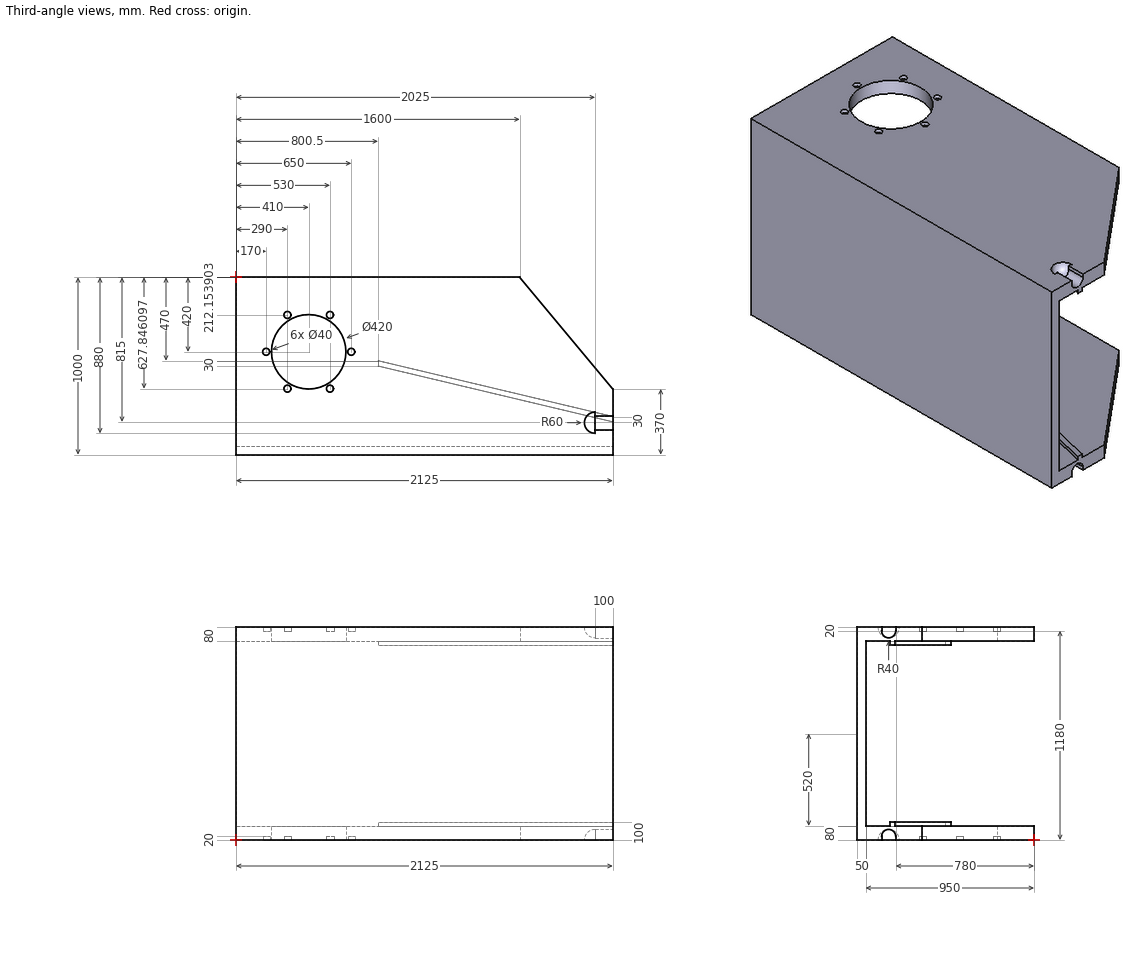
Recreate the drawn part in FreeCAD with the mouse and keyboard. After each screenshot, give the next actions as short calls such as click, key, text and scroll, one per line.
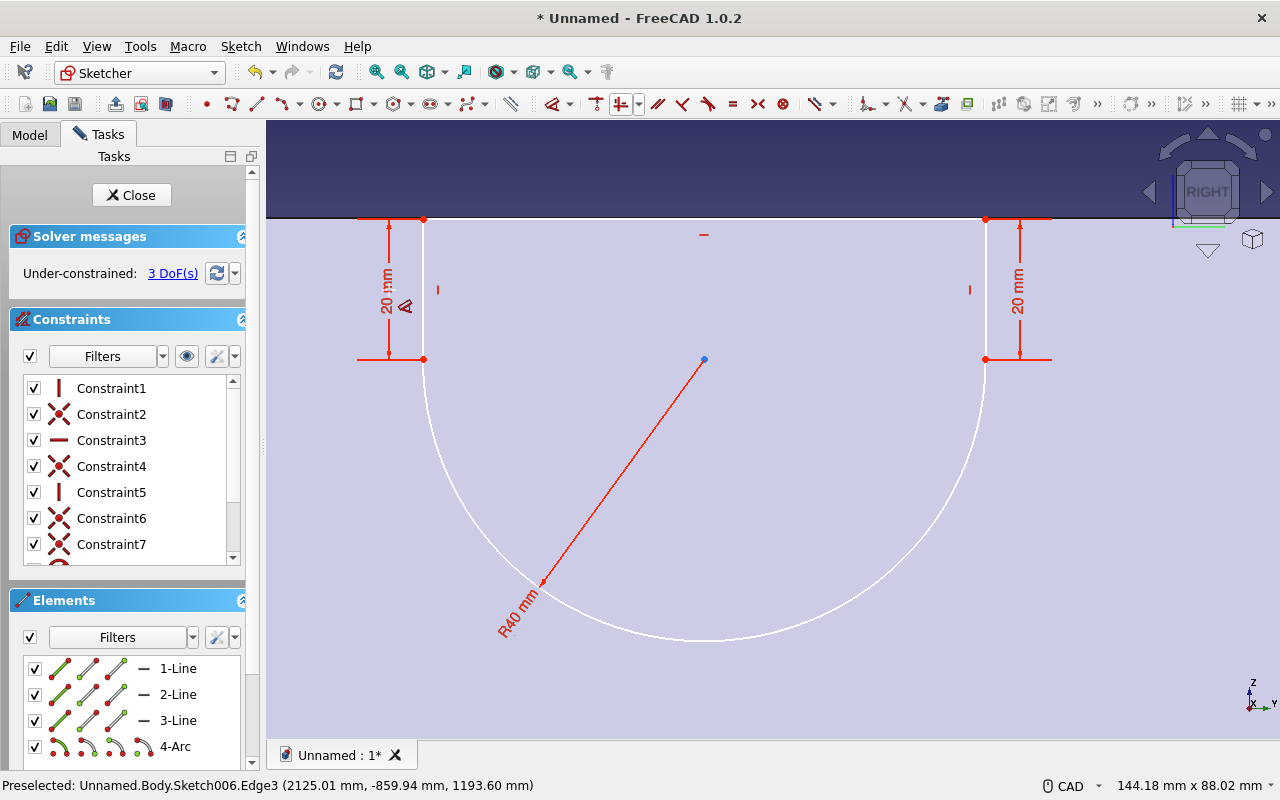
click(986, 360)
click(1050, 326)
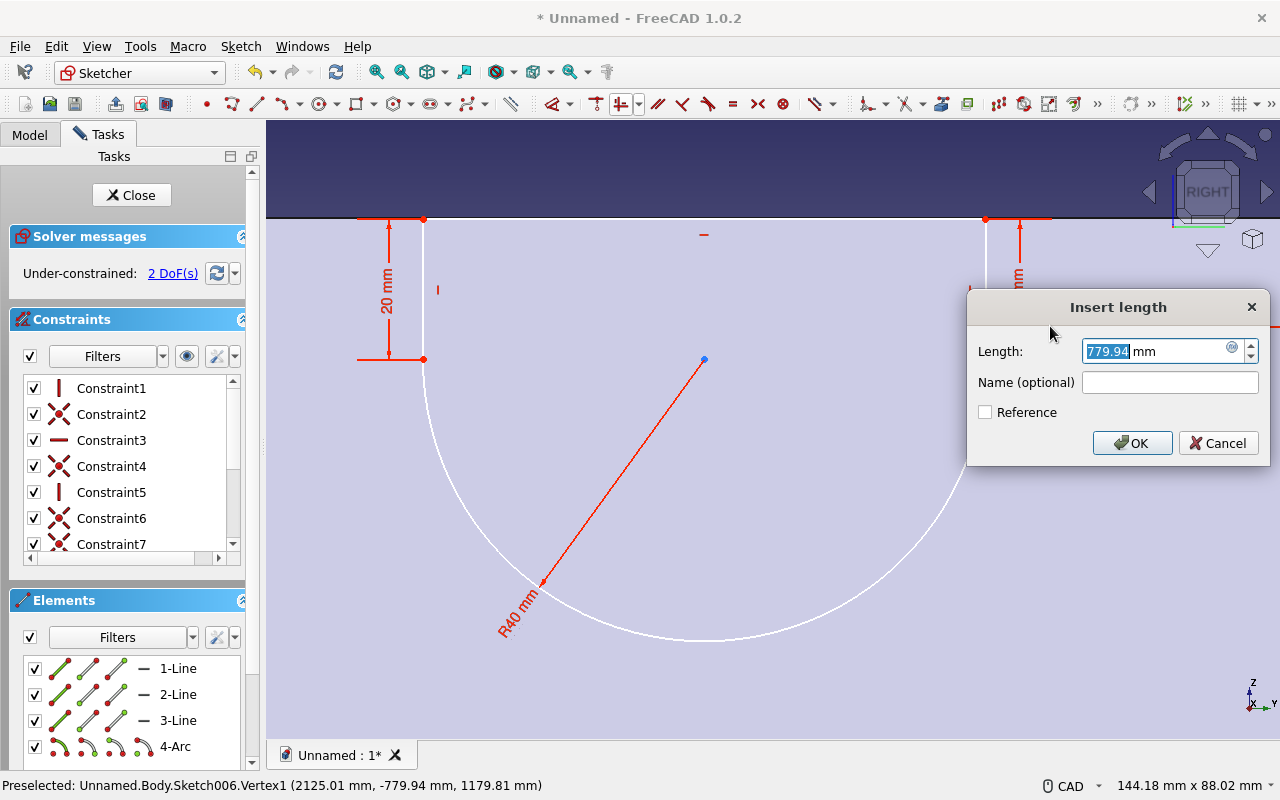
text(780)
key(Return)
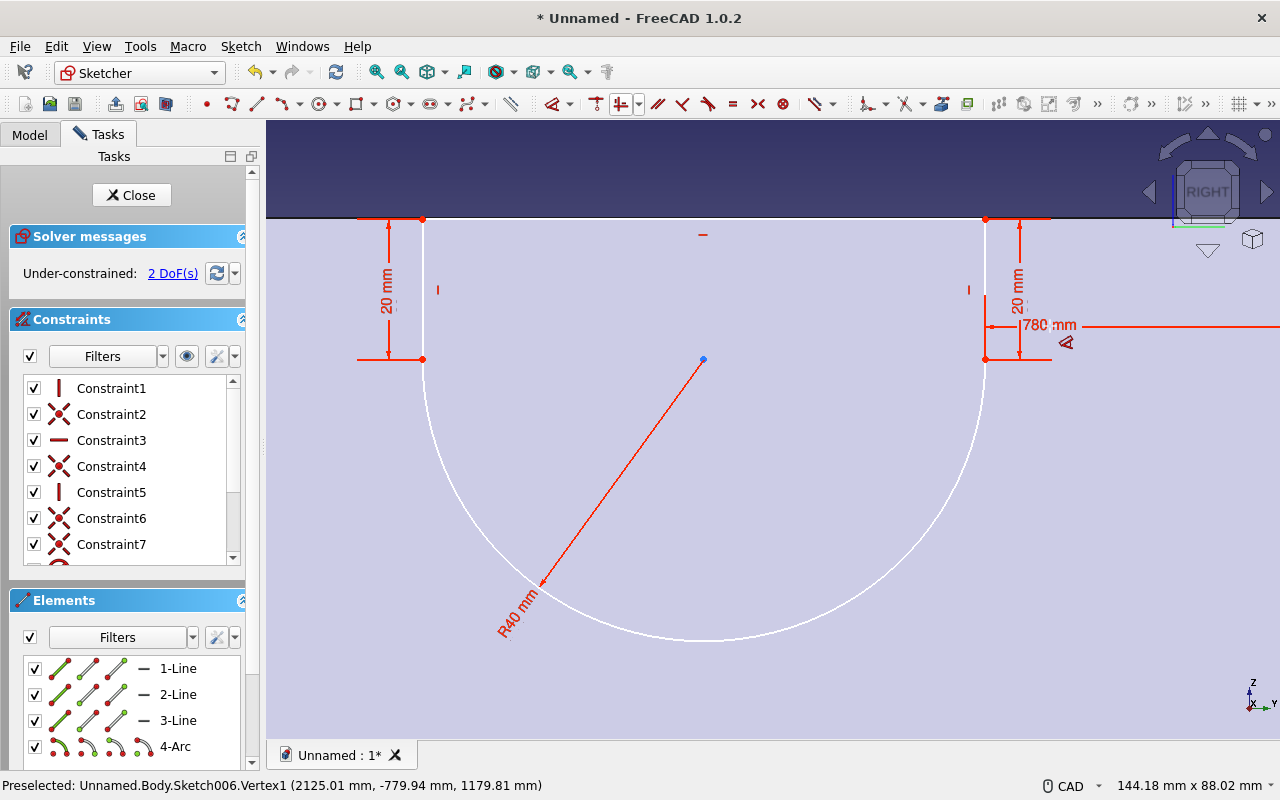
click(985, 360)
click(951, 536)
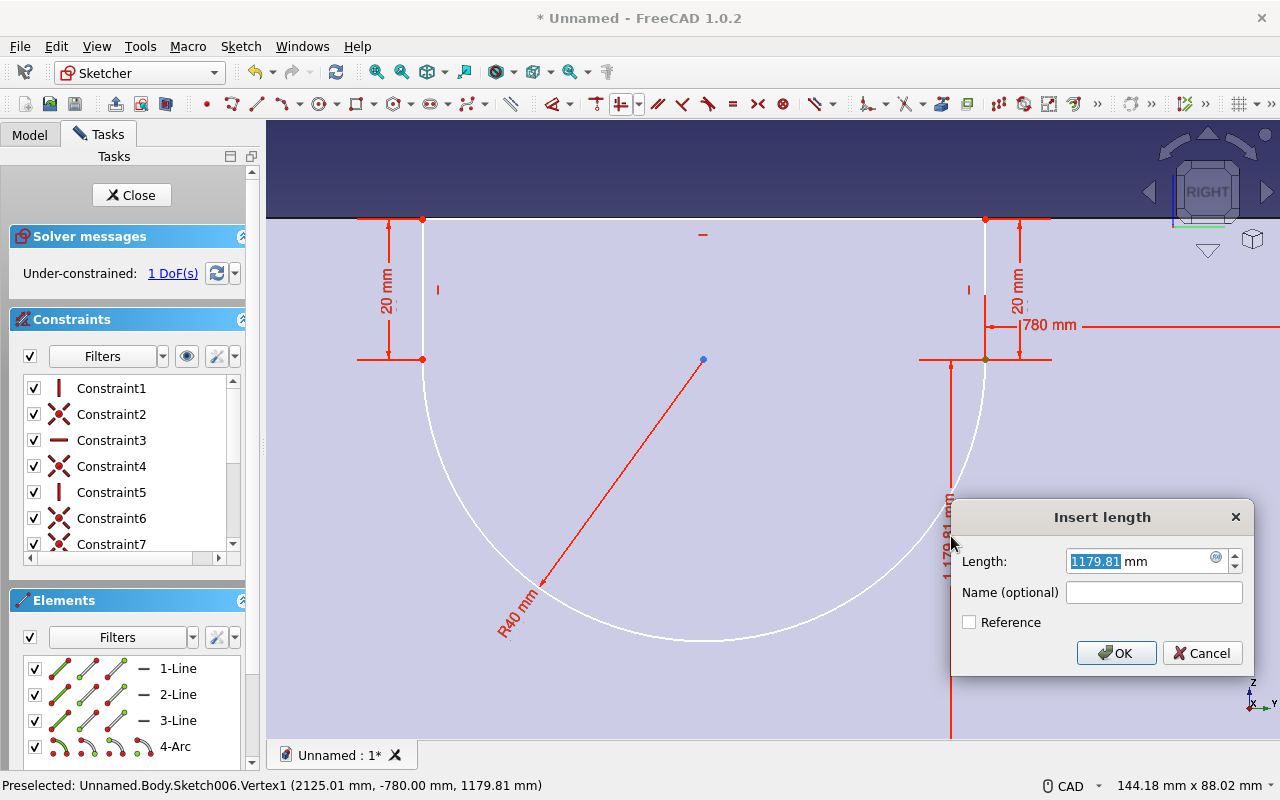
text(1180)
key(Return)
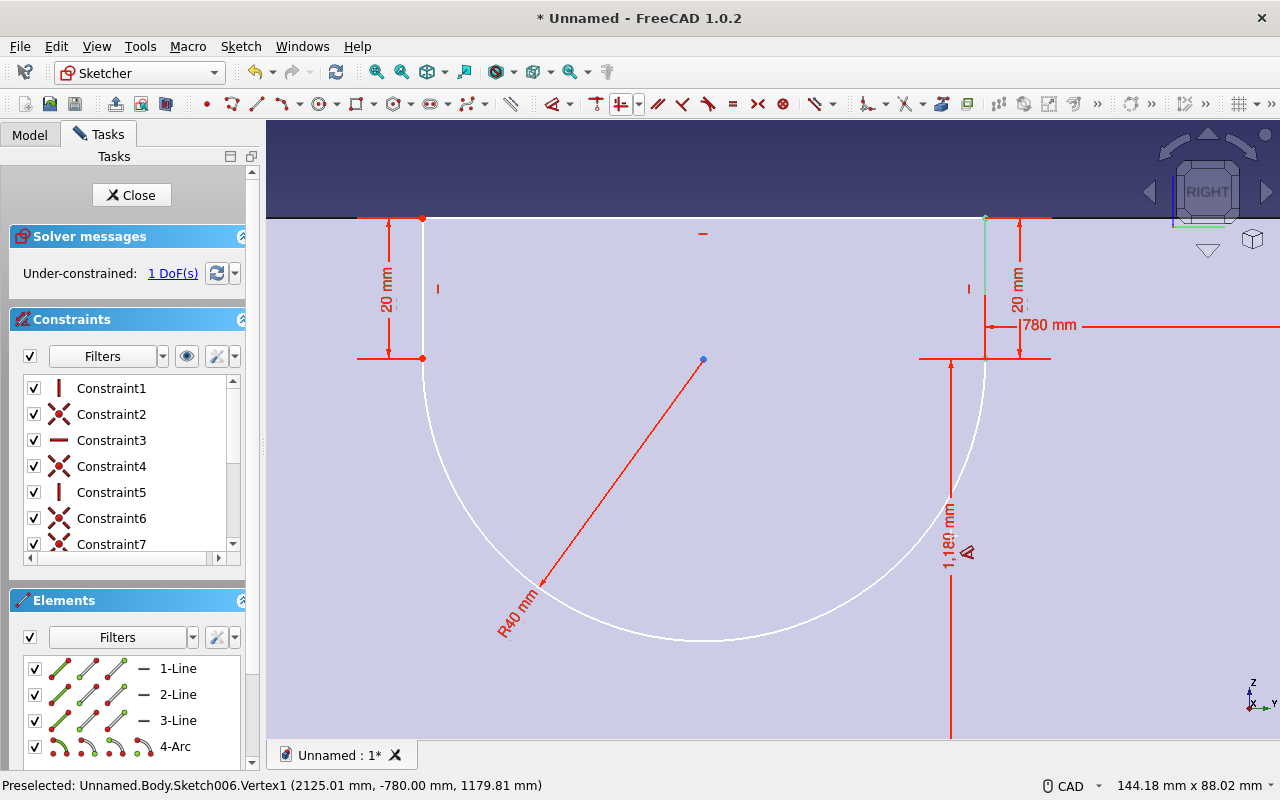
click(704, 360)
click(670, 536)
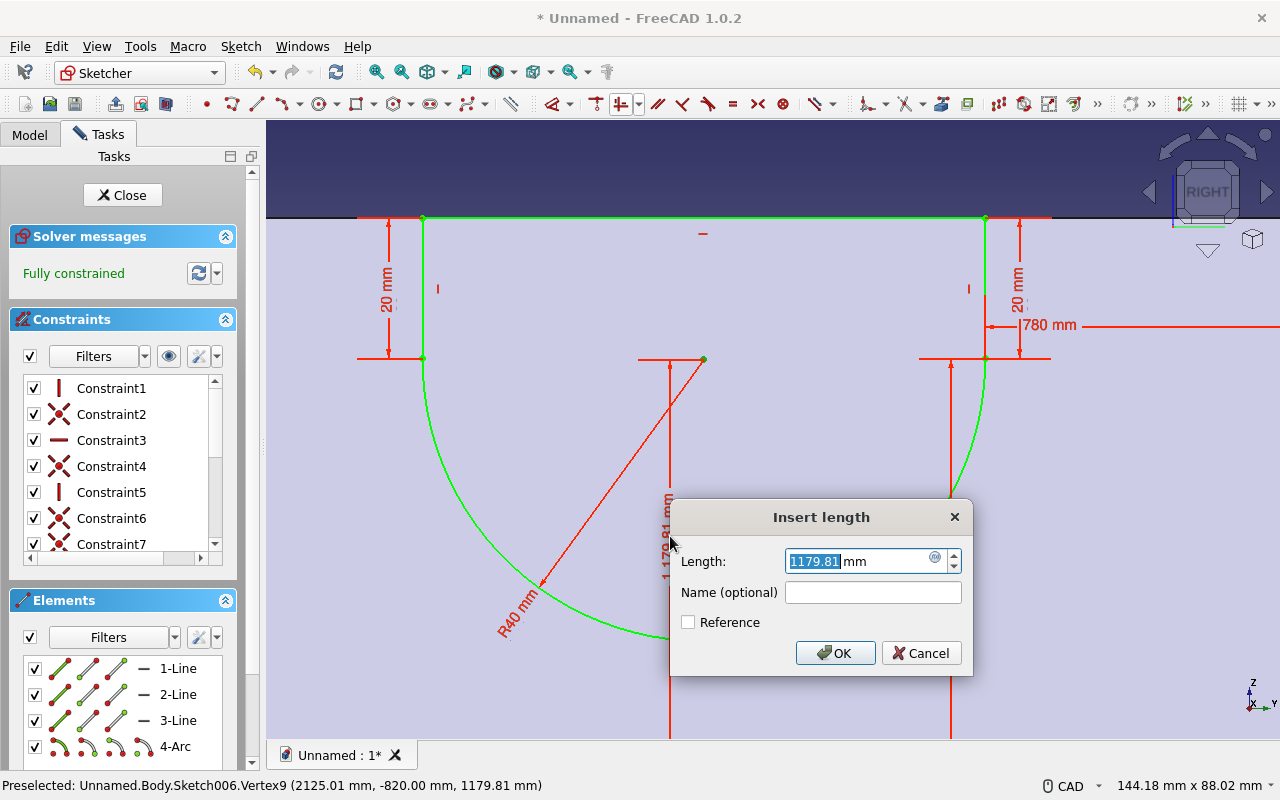
text(1180)
key(Return)
key(Escape)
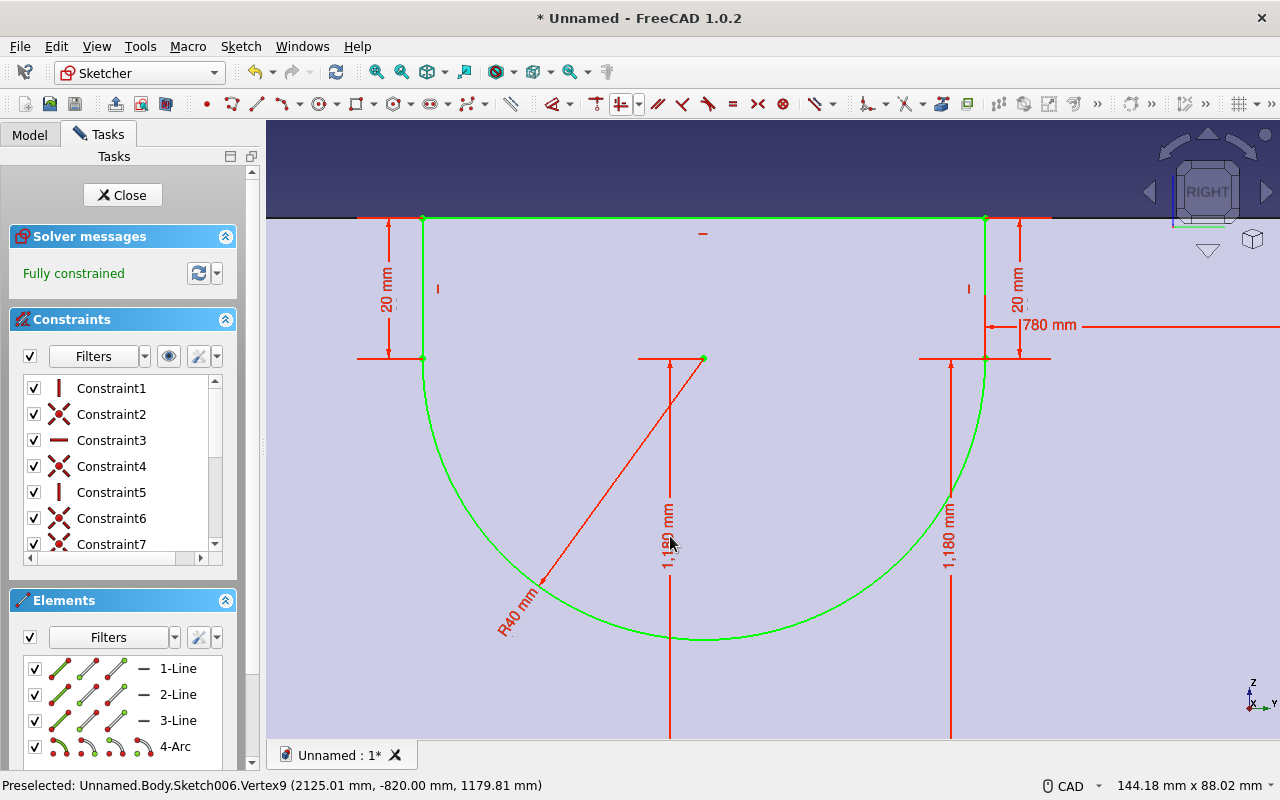
click(123, 195)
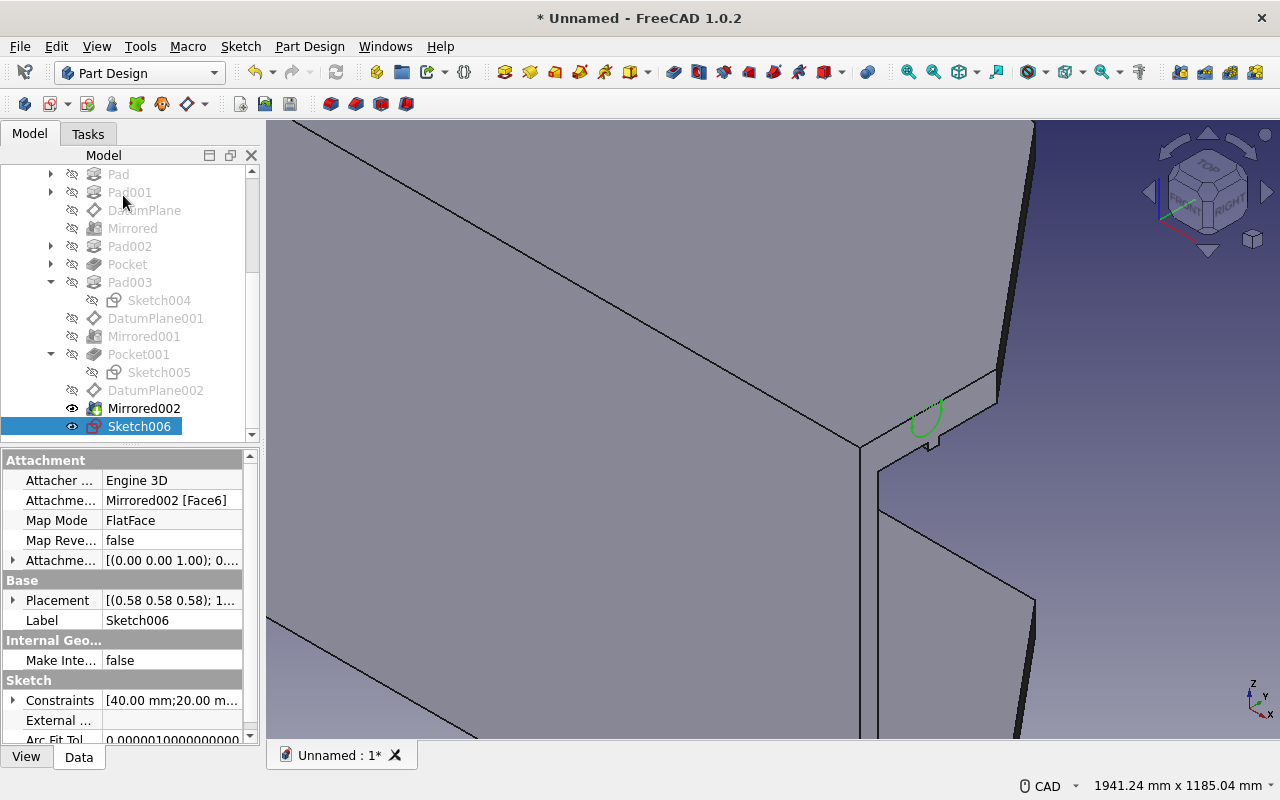
click(674, 72)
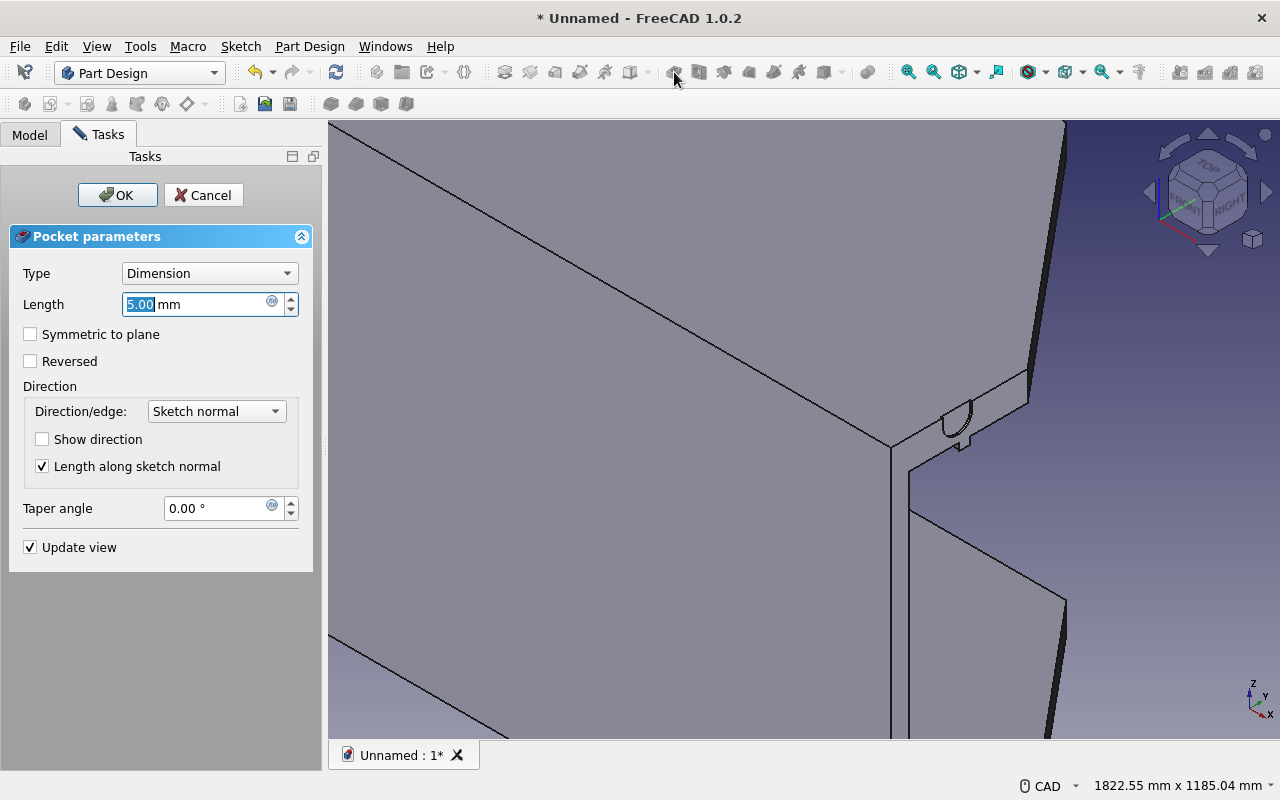
text(100)
key(Tab)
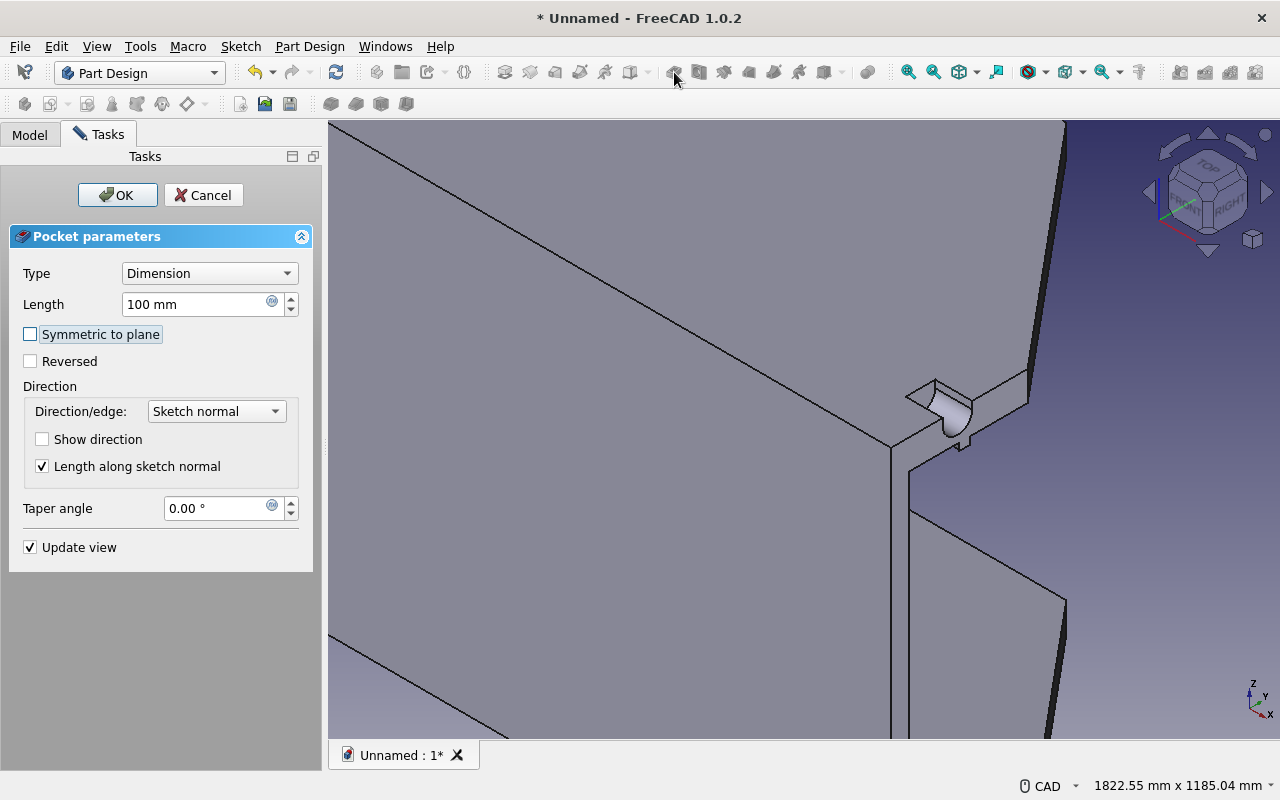
click(118, 195)